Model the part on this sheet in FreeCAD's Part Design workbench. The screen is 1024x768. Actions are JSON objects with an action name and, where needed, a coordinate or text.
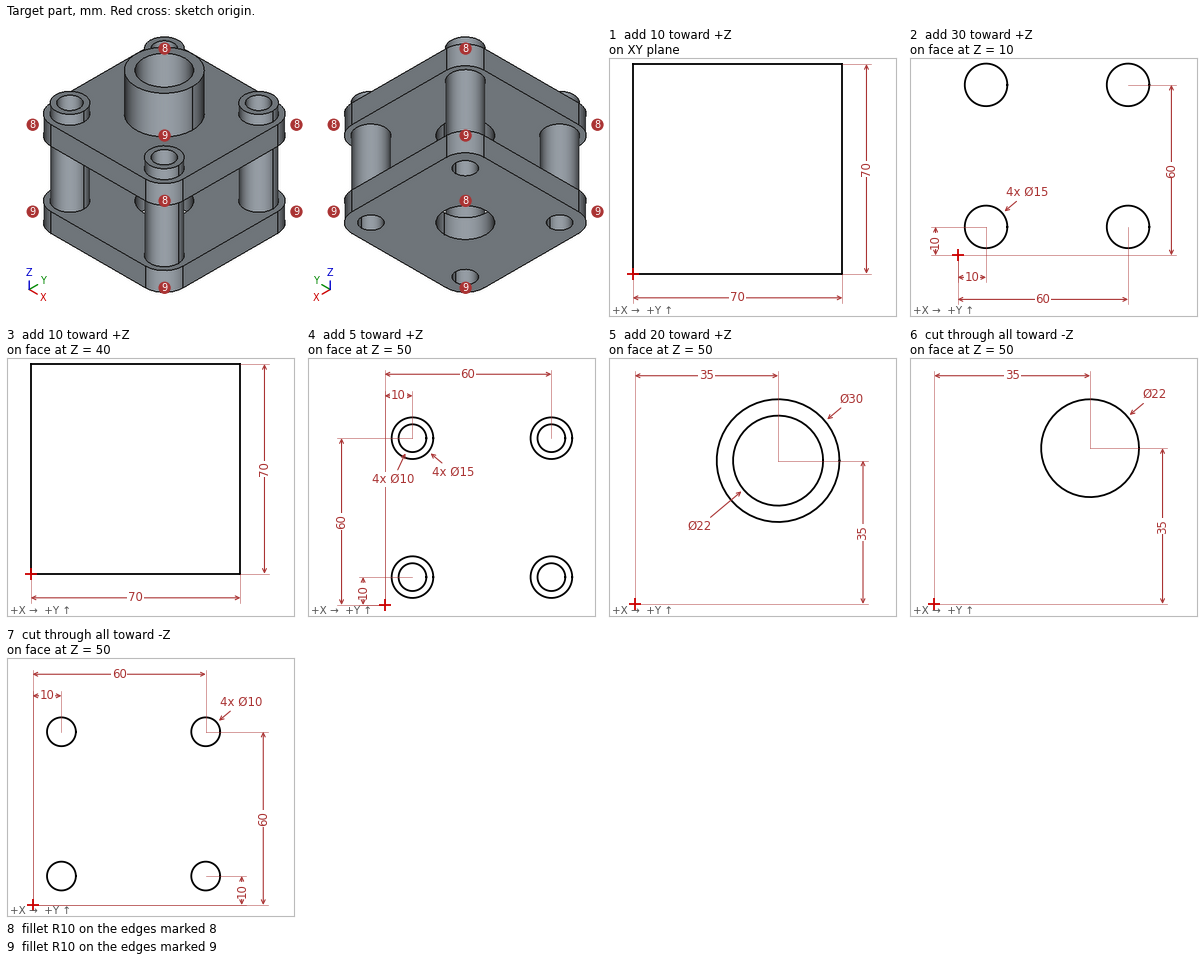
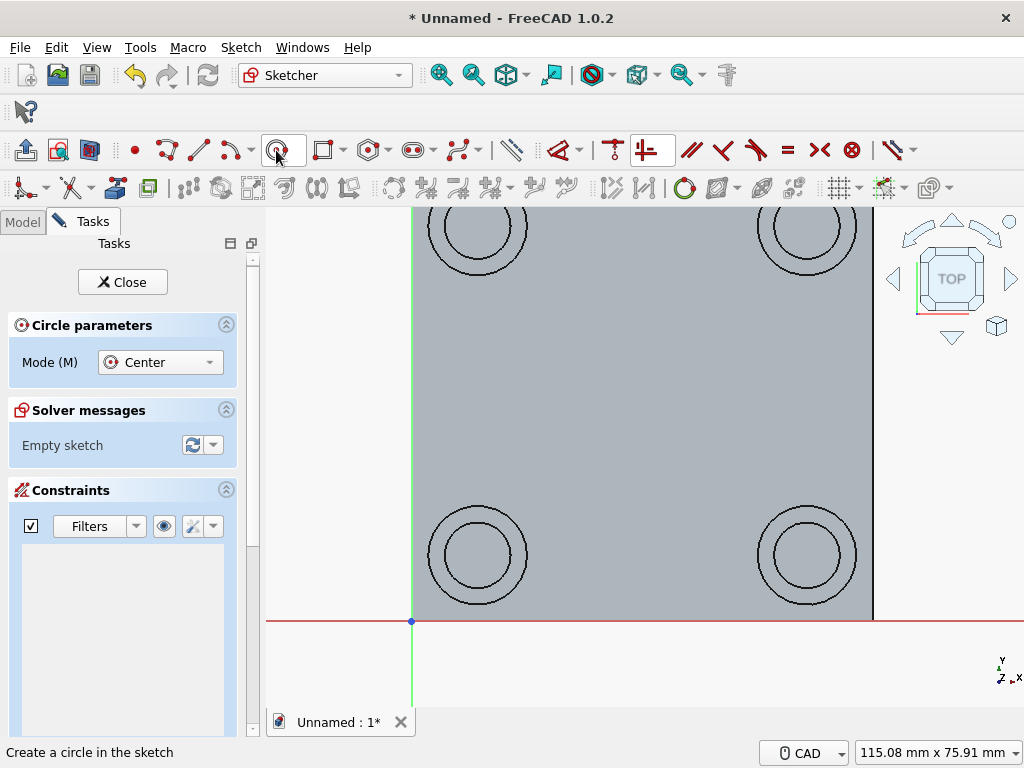
{"action": "left_click", "coordinate": [642, 391]}
{"action": "left_click", "coordinate": [712, 321]}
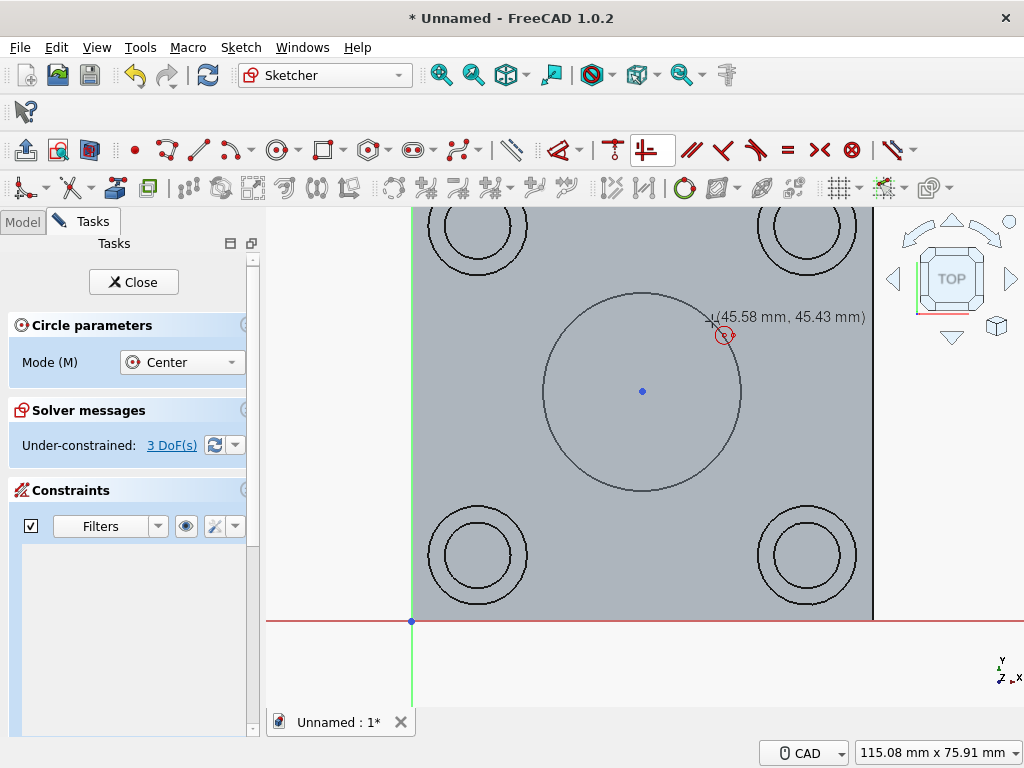
{"action": "left_click", "coordinate": [642, 392]}
{"action": "left_click", "coordinate": [694, 339]}
{"action": "key", "text": "Escape"}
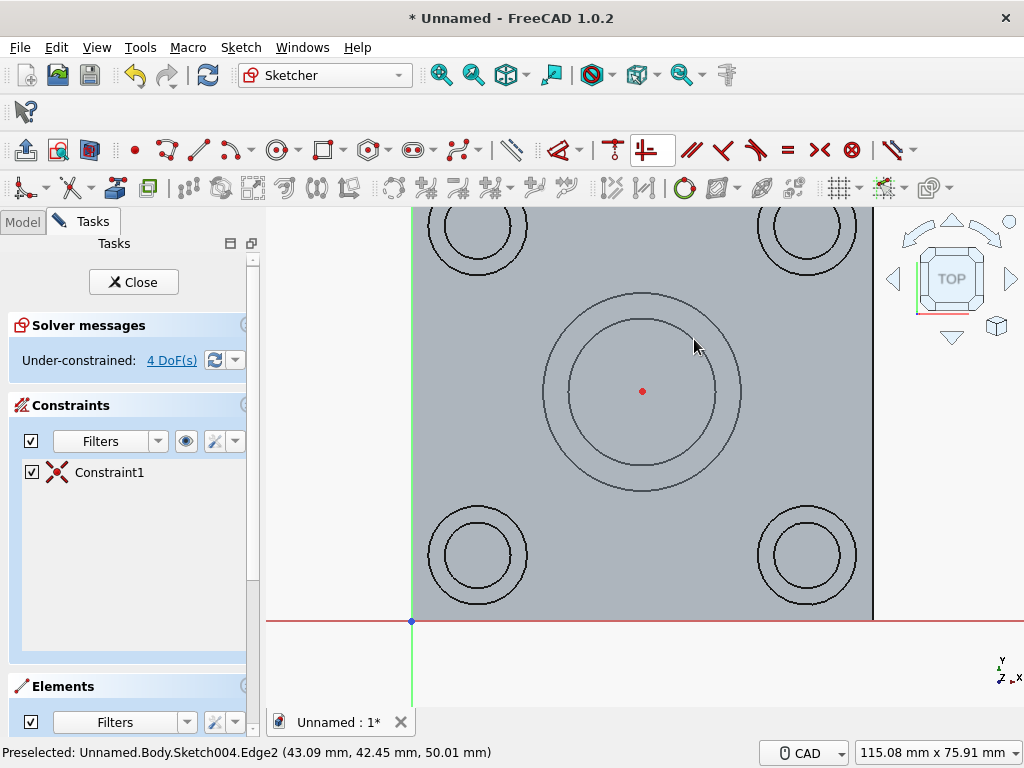
{"action": "key", "text": "d"}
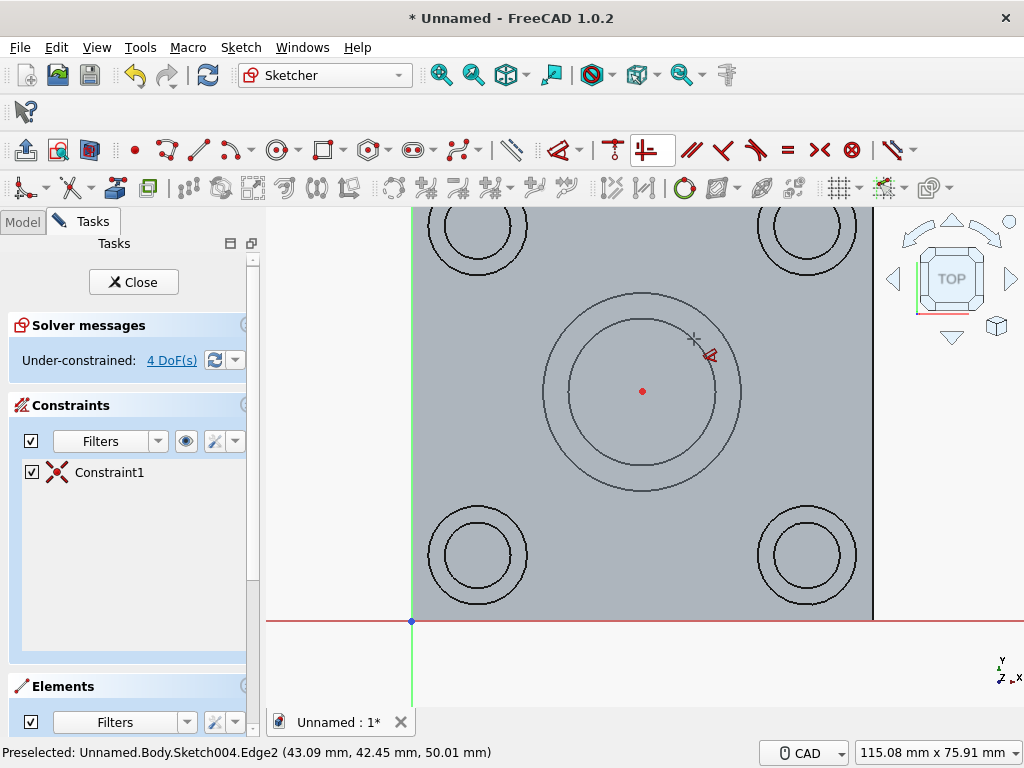
{"action": "left_click", "coordinate": [712, 322]}
{"action": "left_click", "coordinate": [735, 299]}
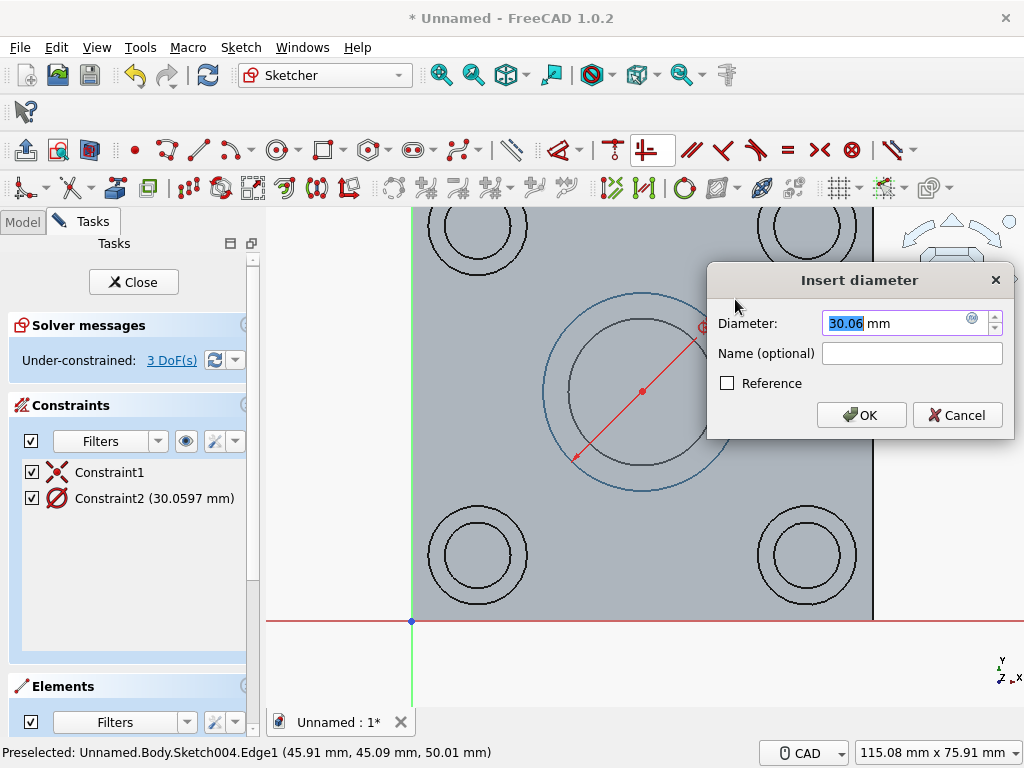
{"action": "type", "text": "30"}
{"action": "key", "text": "Return"}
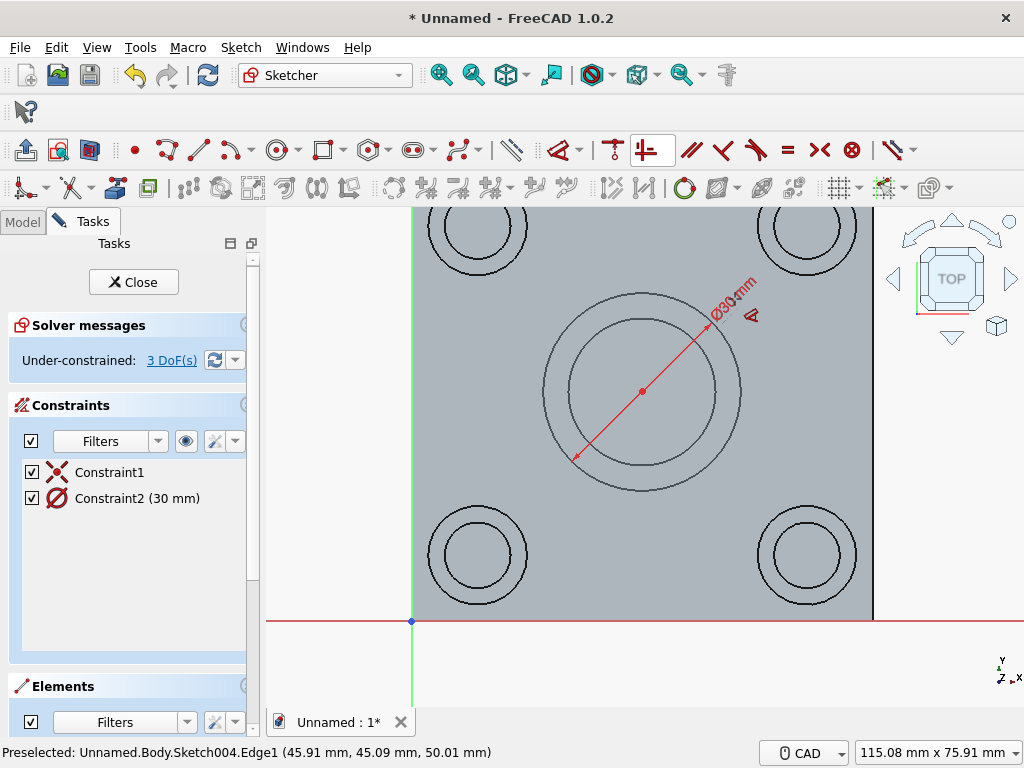
{"action": "left_click", "coordinate": [694, 340]}
{"action": "left_click", "coordinate": [765, 356]}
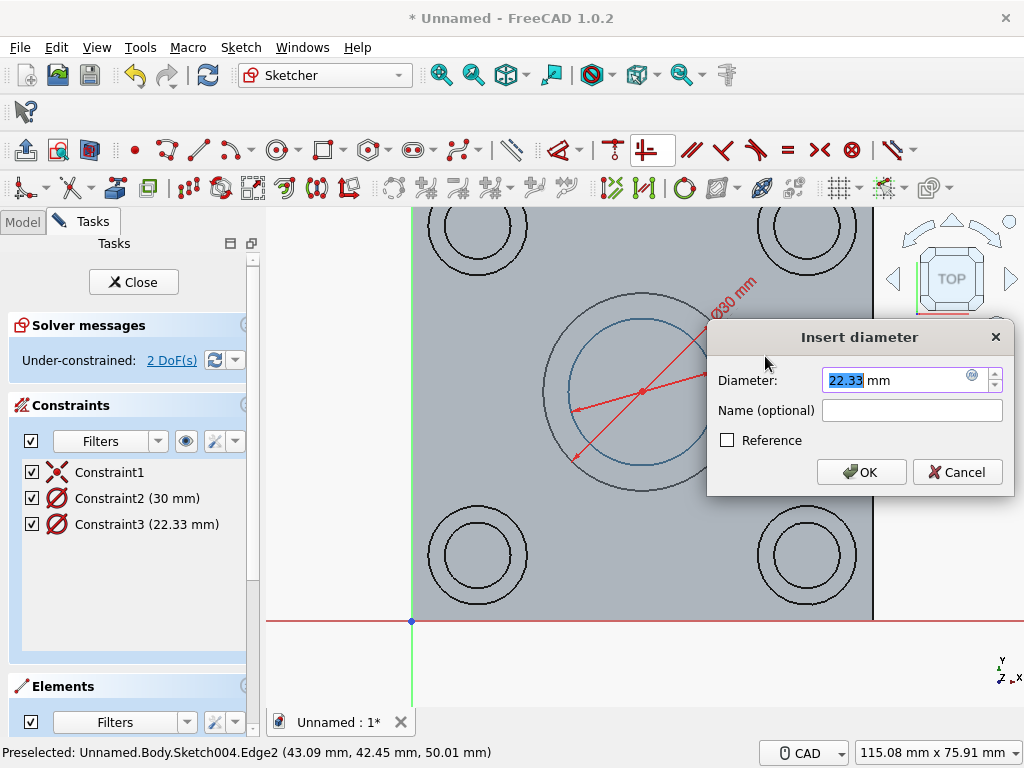
{"action": "type", "text": "22"}
{"action": "key", "text": "Return"}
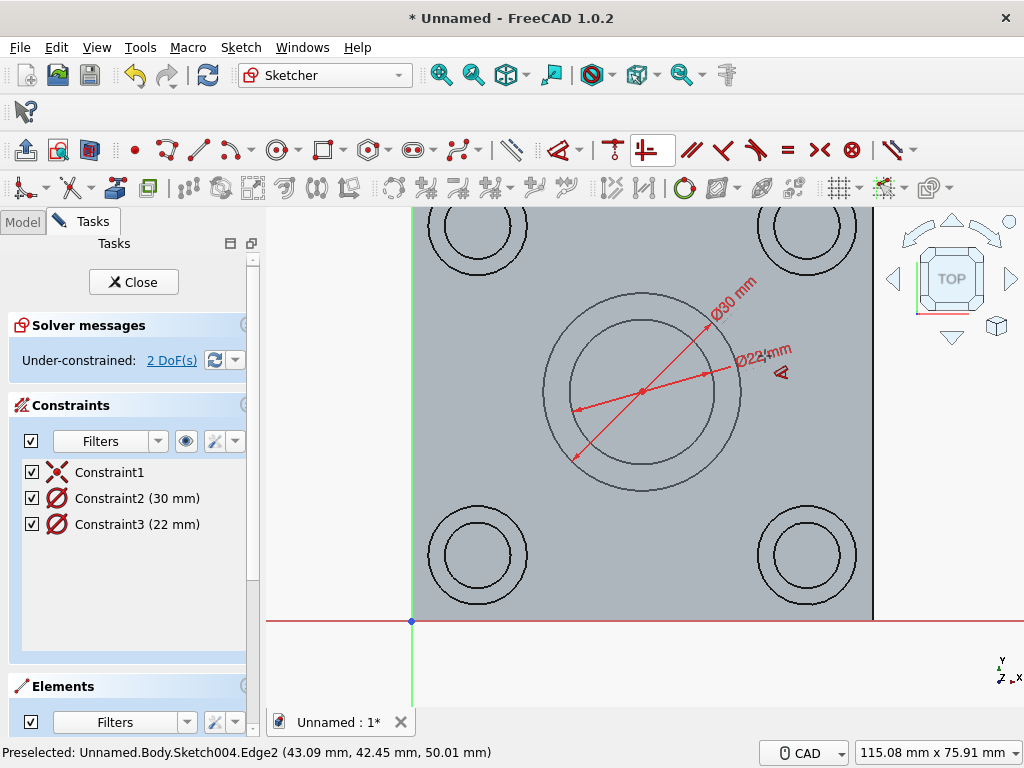
{"action": "left_click", "coordinate": [642, 392]}
{"action": "left_click", "coordinate": [527, 655]}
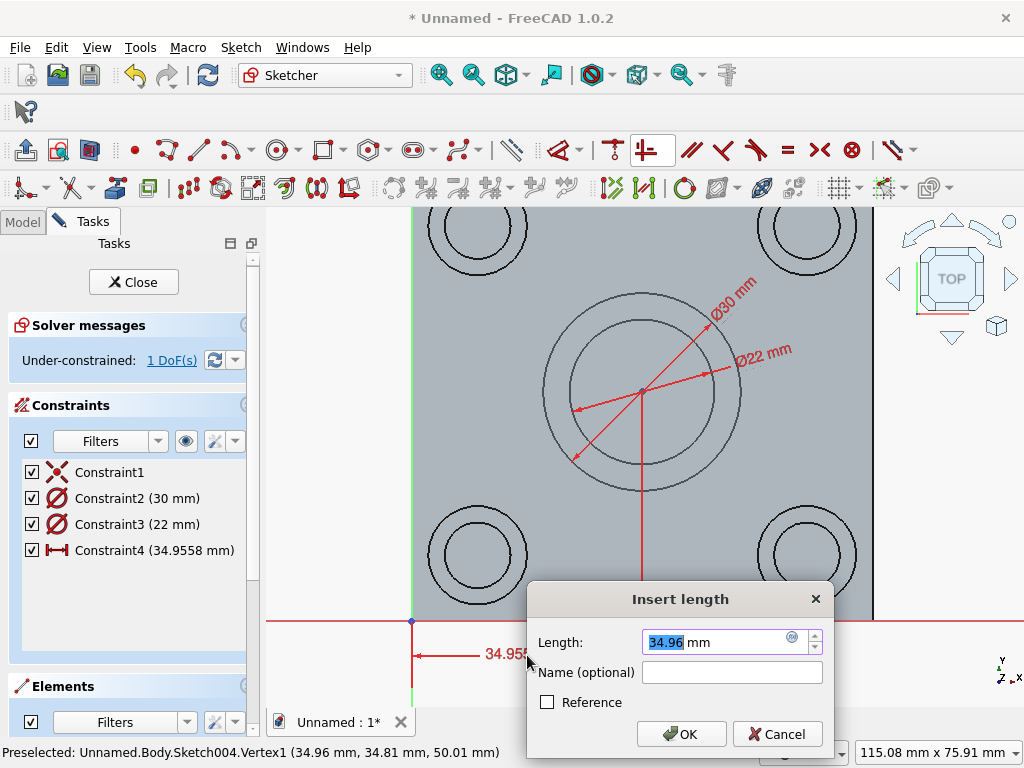
{"action": "type", "text": "35"}
{"action": "key", "text": "Return"}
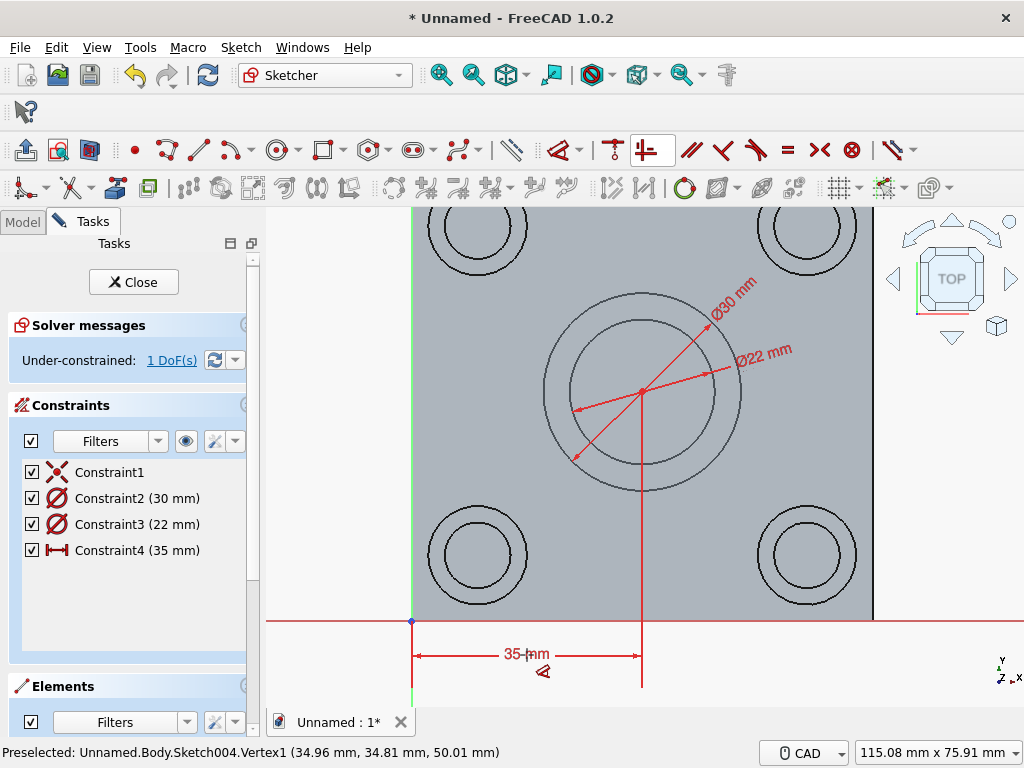
{"action": "left_click", "coordinate": [642, 392]}
{"action": "left_click", "coordinate": [378, 507]}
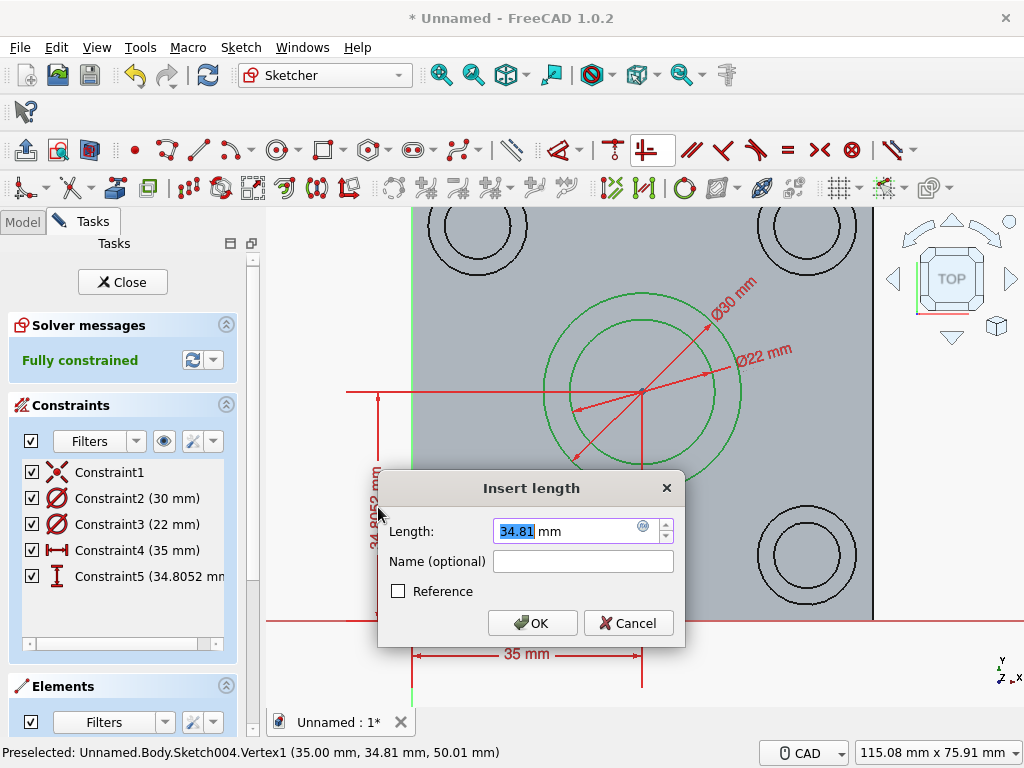
{"action": "type", "text": "35"}
{"action": "key", "text": "Return"}
{"action": "key", "text": "Escape"}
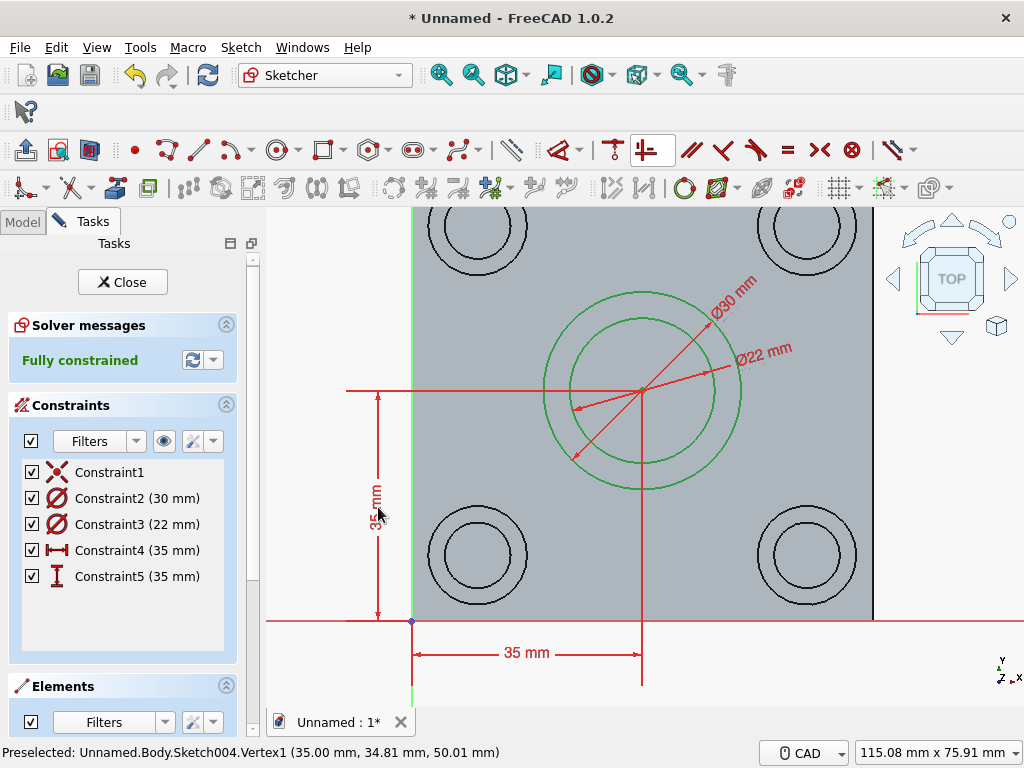
{"action": "left_click", "coordinate": [123, 282]}